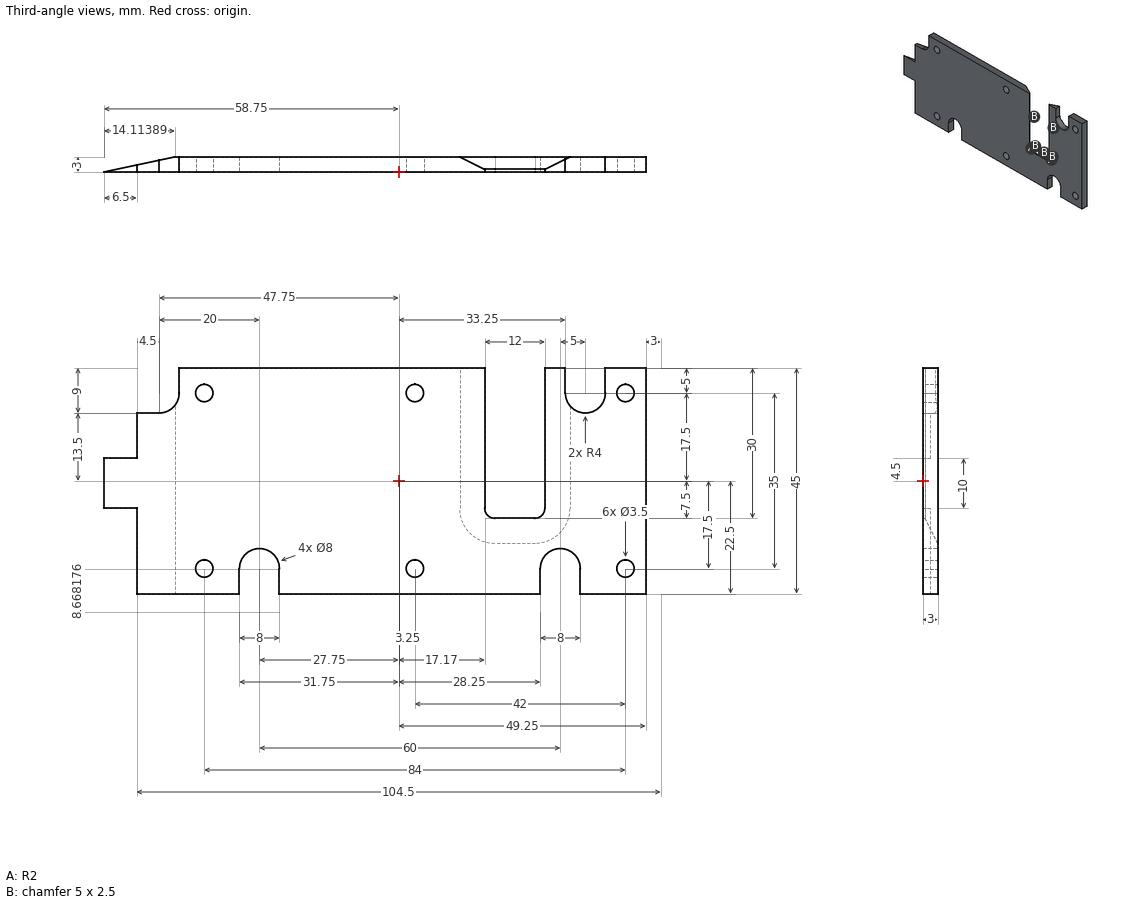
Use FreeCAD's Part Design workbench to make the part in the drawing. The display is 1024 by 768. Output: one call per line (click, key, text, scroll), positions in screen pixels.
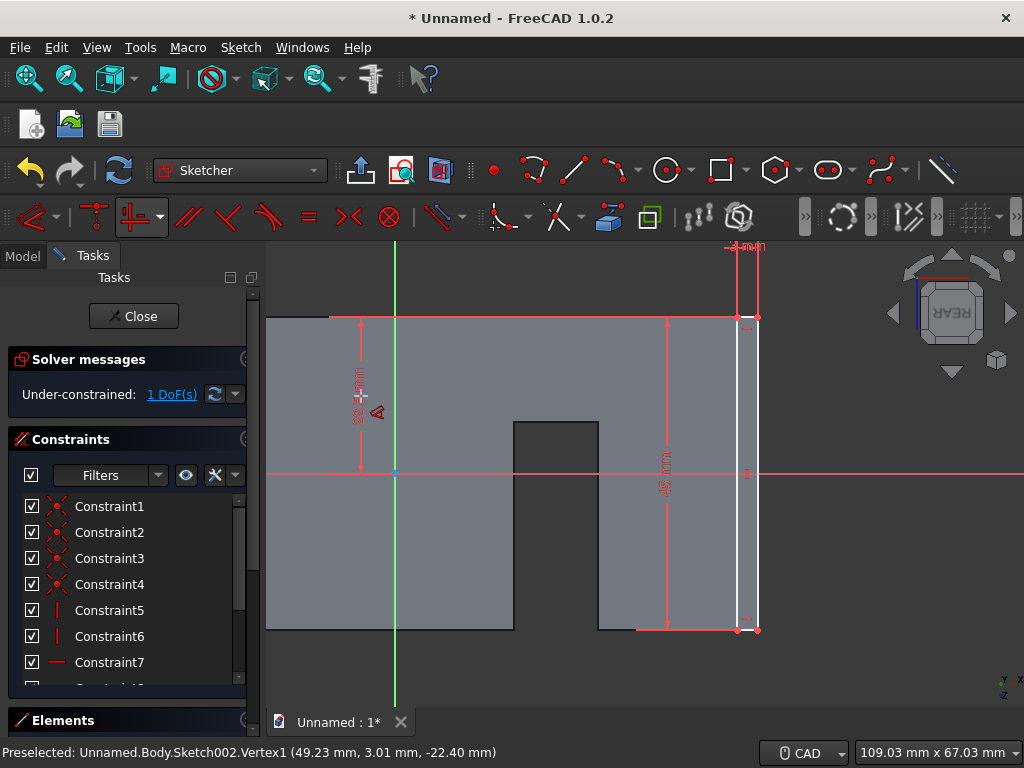
click(737, 317)
click(566, 283)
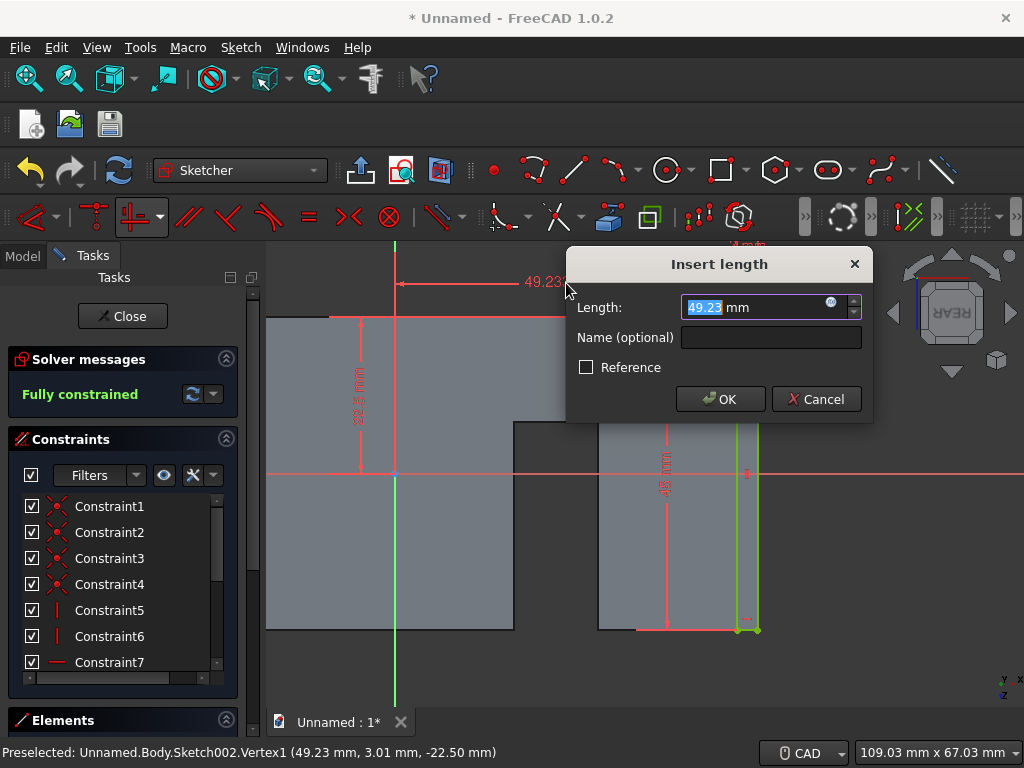
text(49.25)
key(Return)
key(Escape)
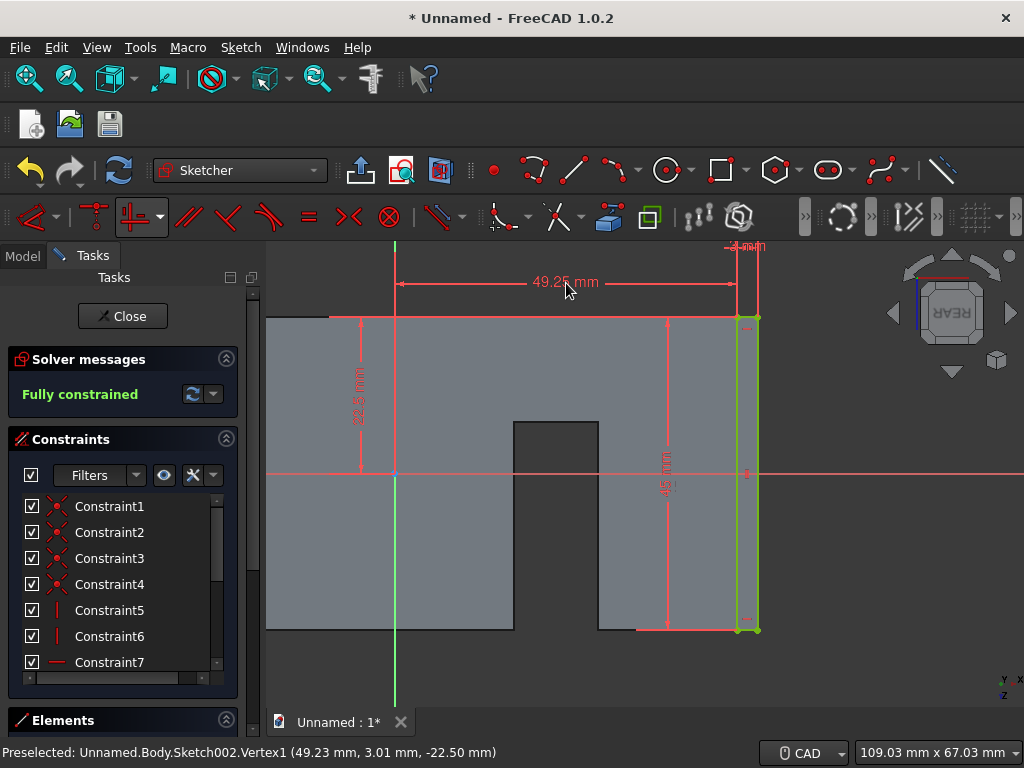
click(123, 316)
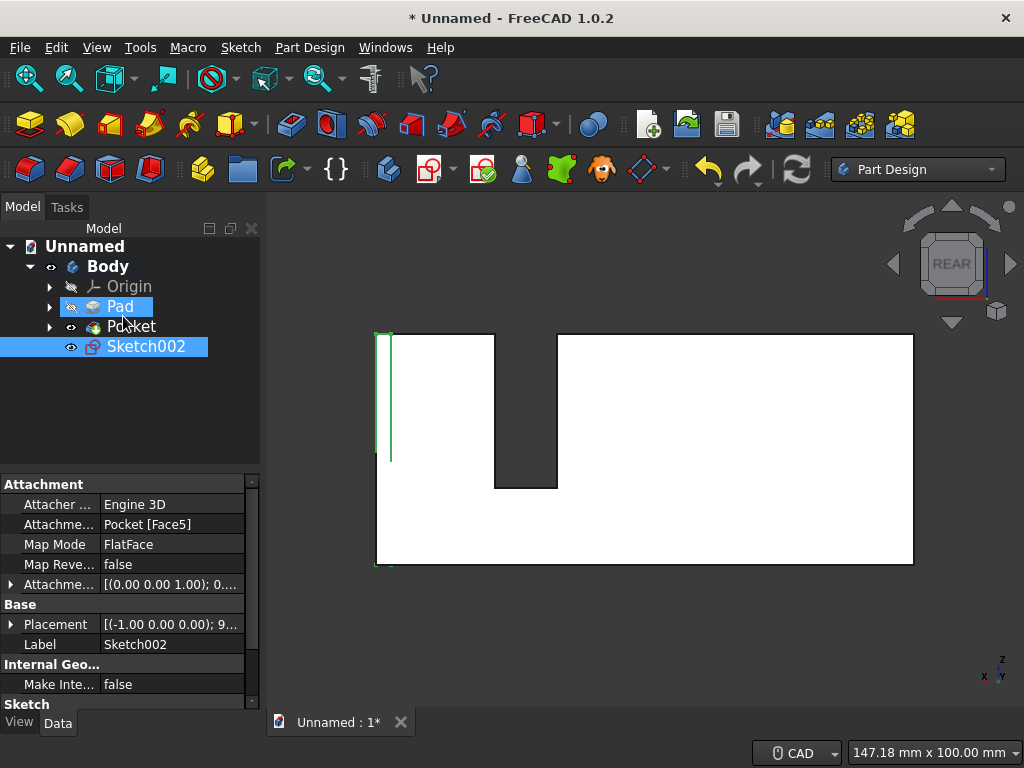
click(292, 124)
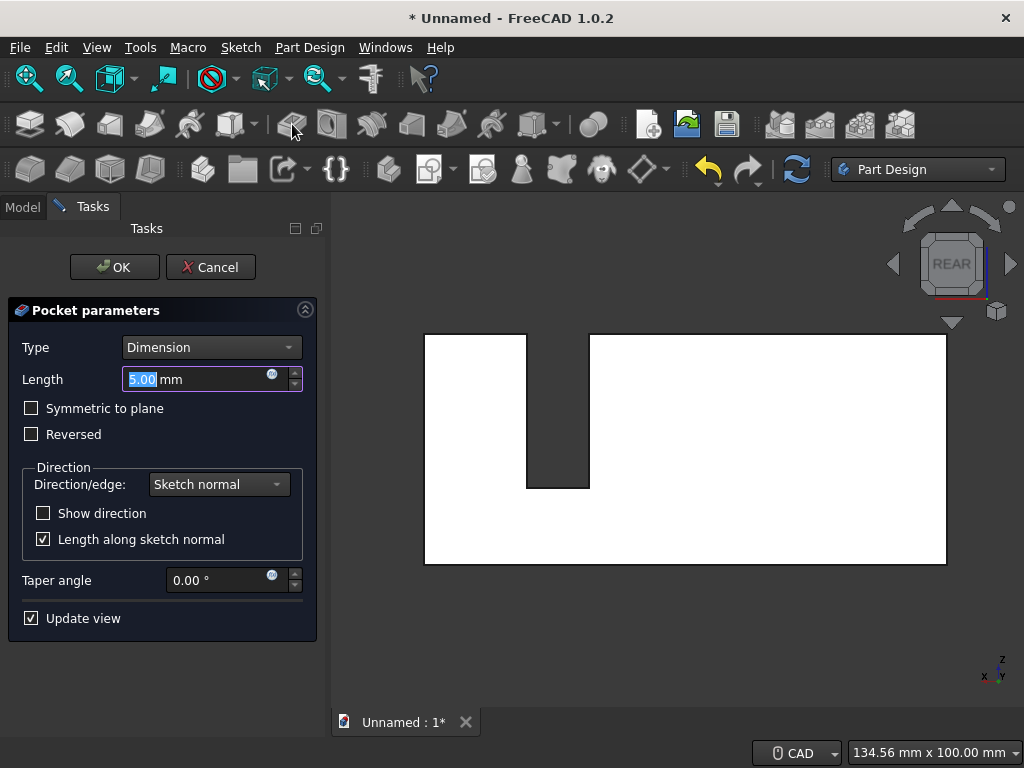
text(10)
key(Tab)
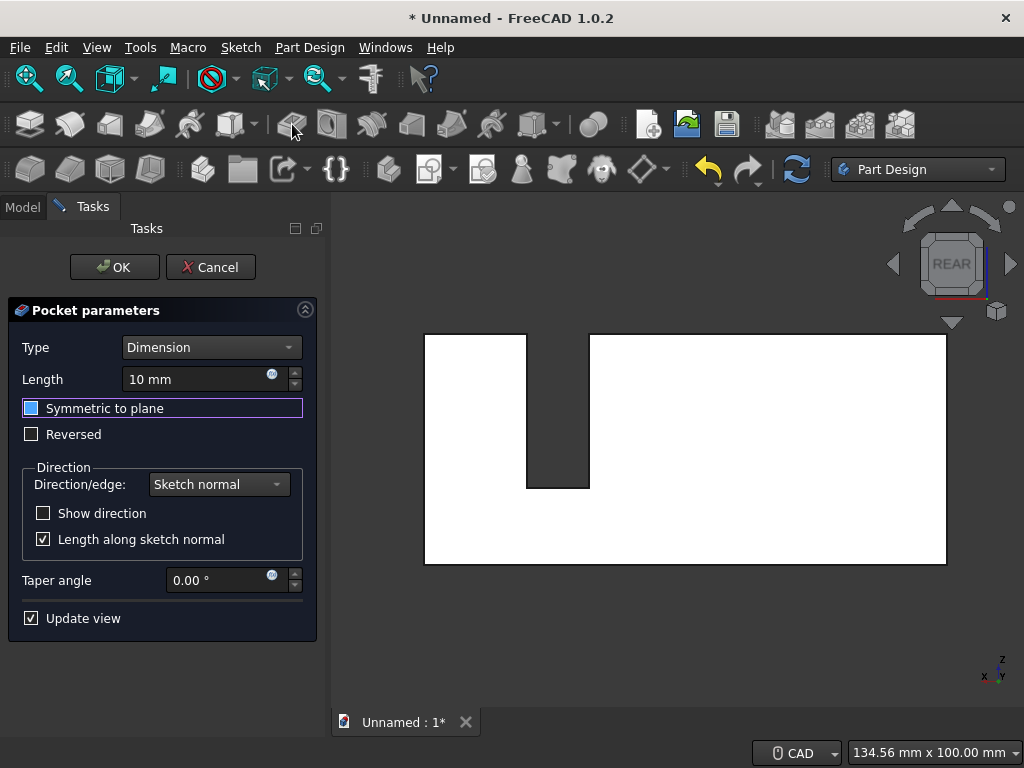
click(115, 267)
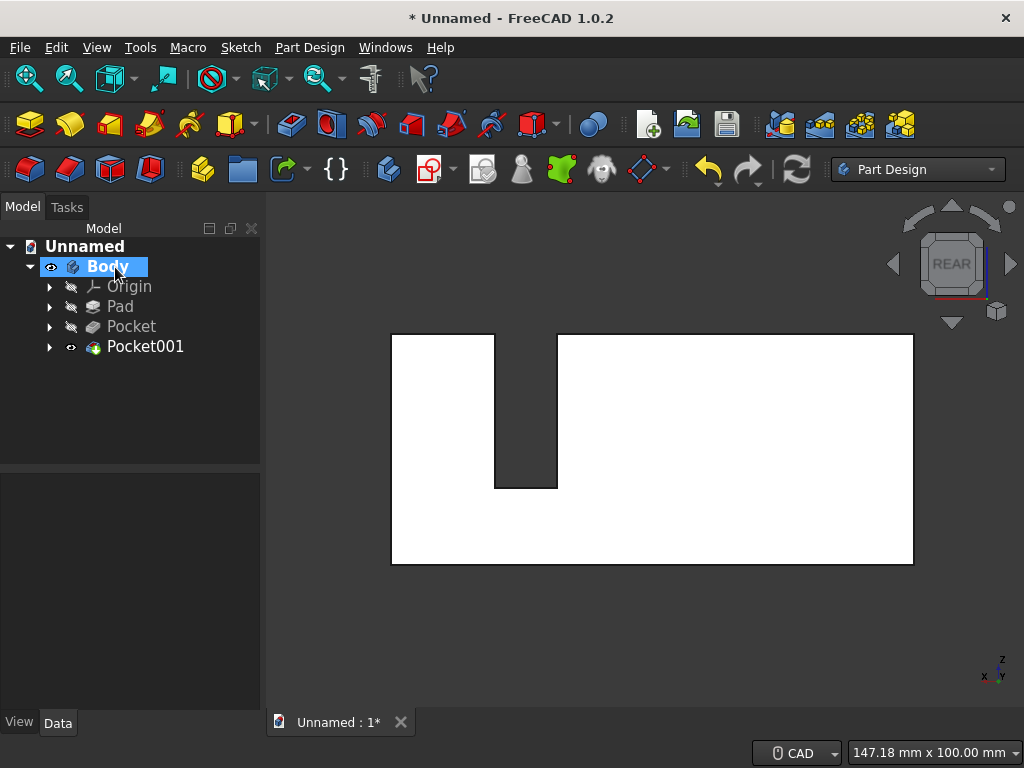
click(727, 448)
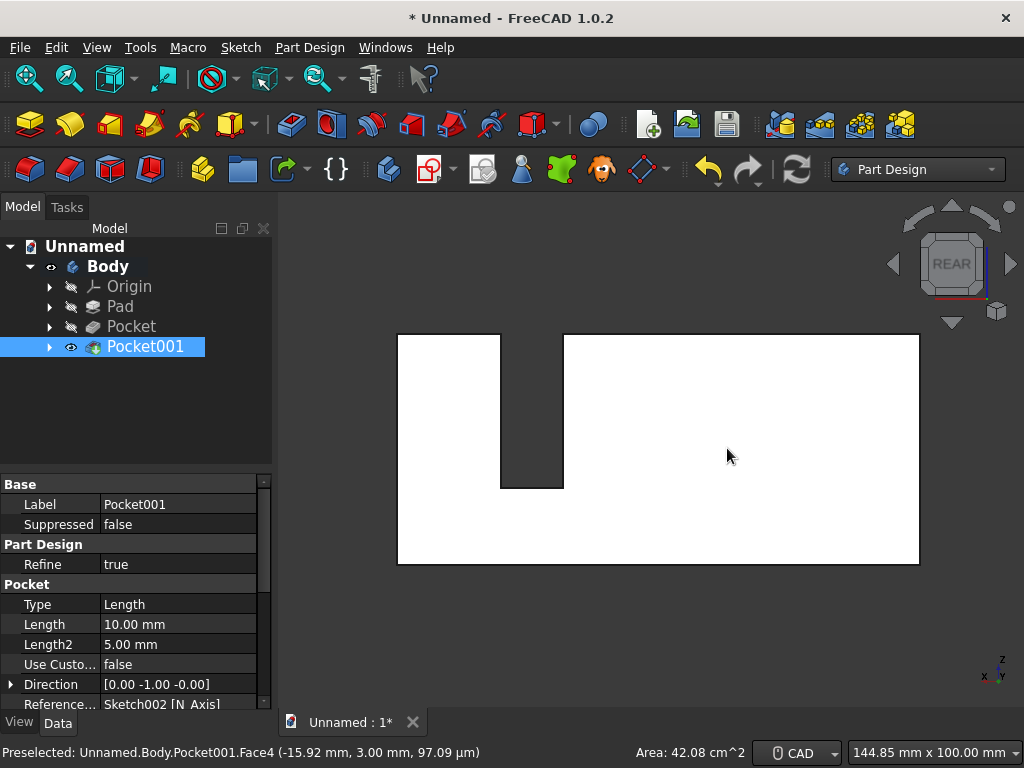
click(430, 170)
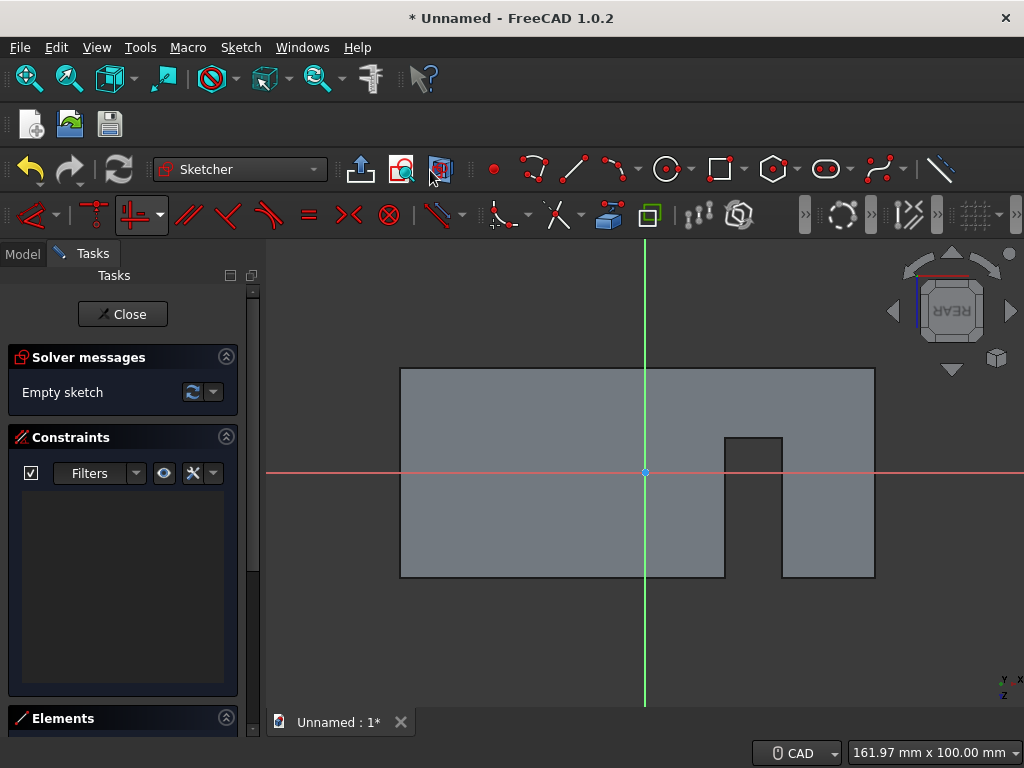
scroll(294, 473, down, 1)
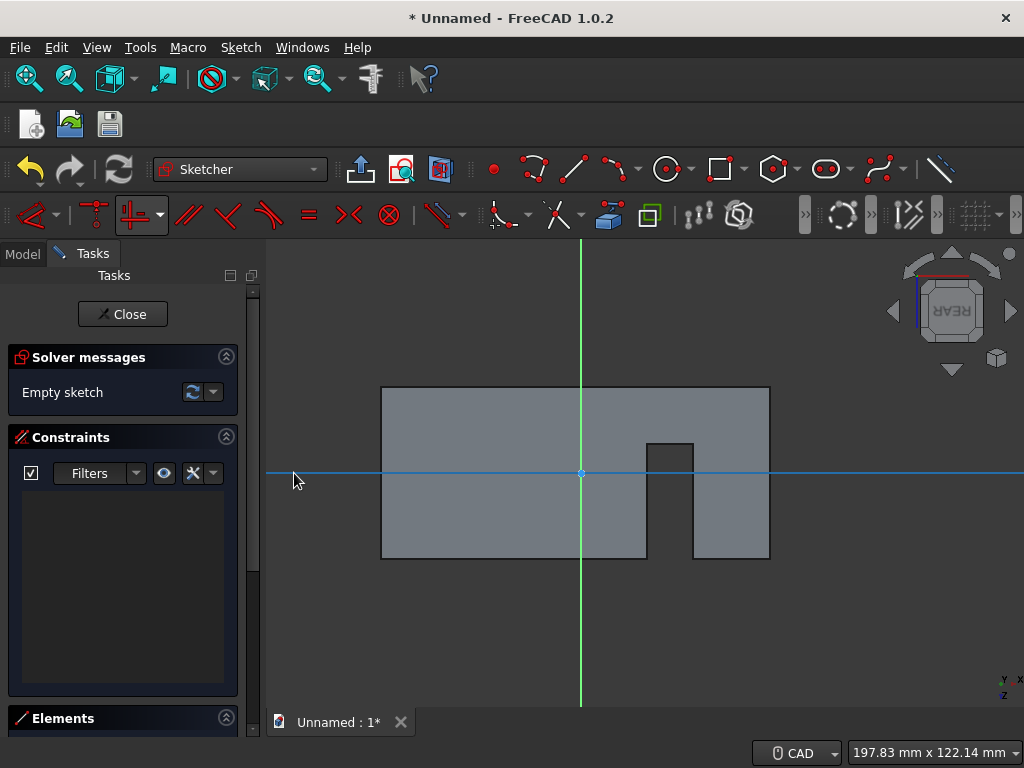
click(668, 170)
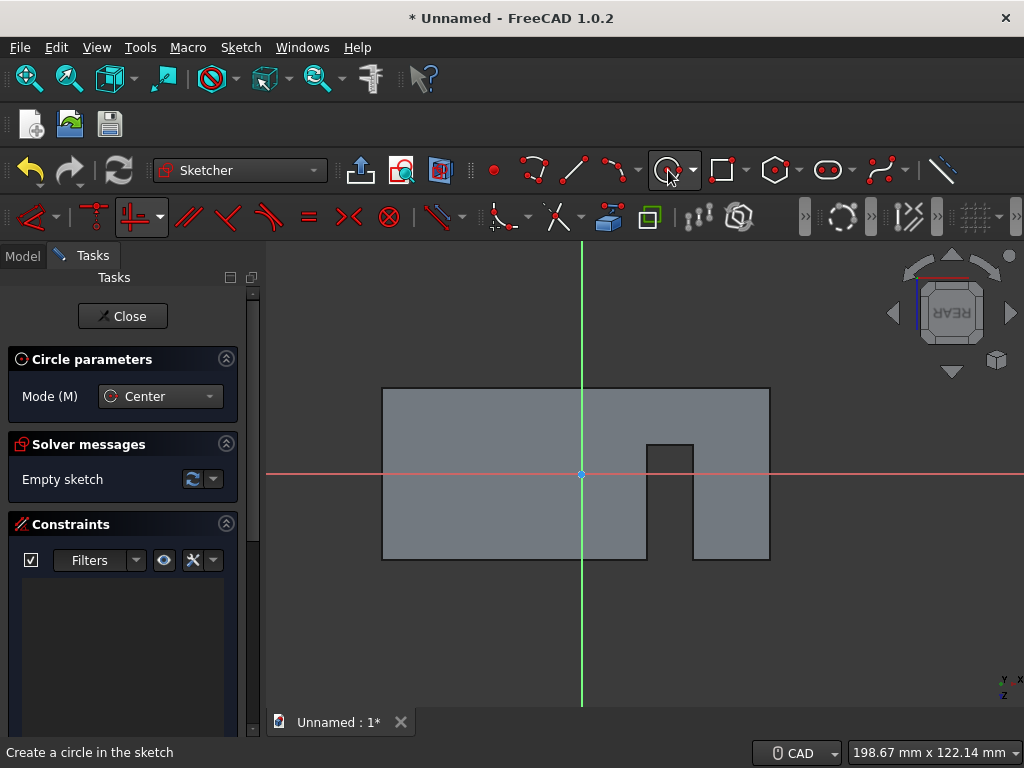
scroll(754, 407, up, 7)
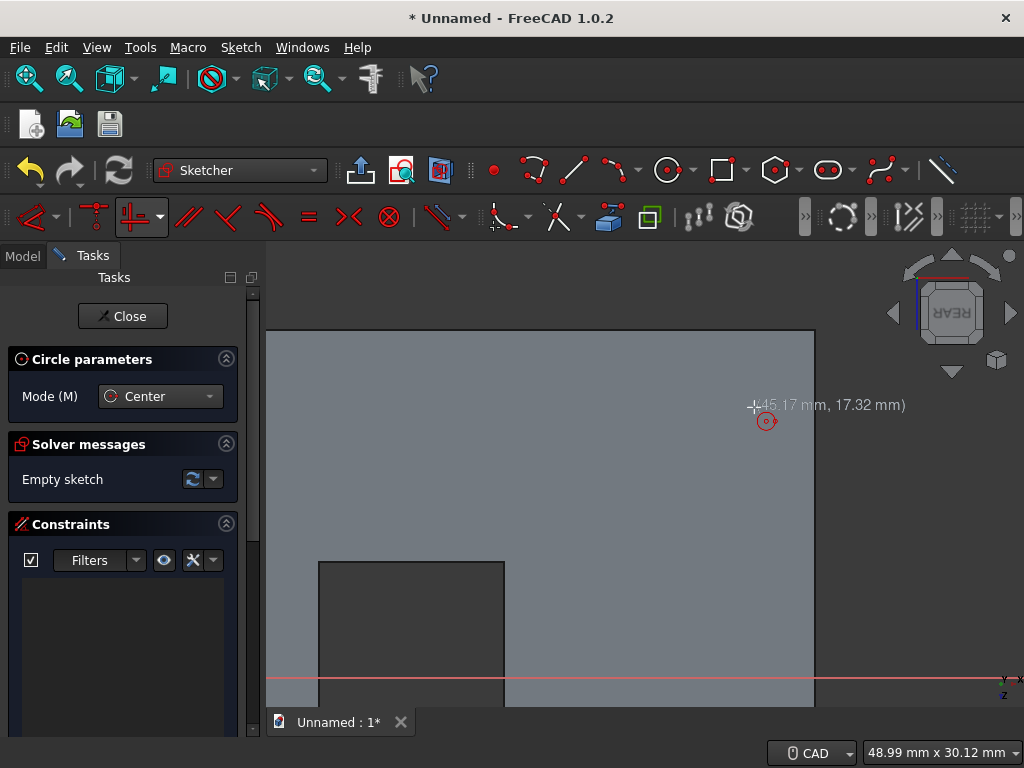
scroll(780, 386, down, 6)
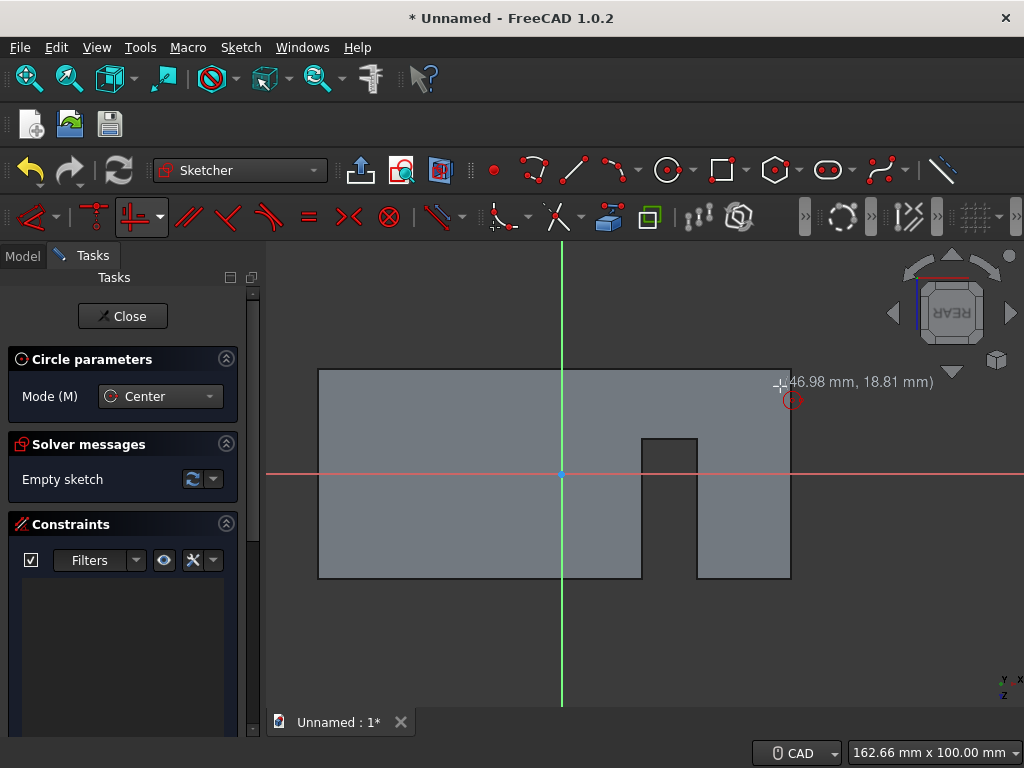
click(772, 393)
move(778, 387)